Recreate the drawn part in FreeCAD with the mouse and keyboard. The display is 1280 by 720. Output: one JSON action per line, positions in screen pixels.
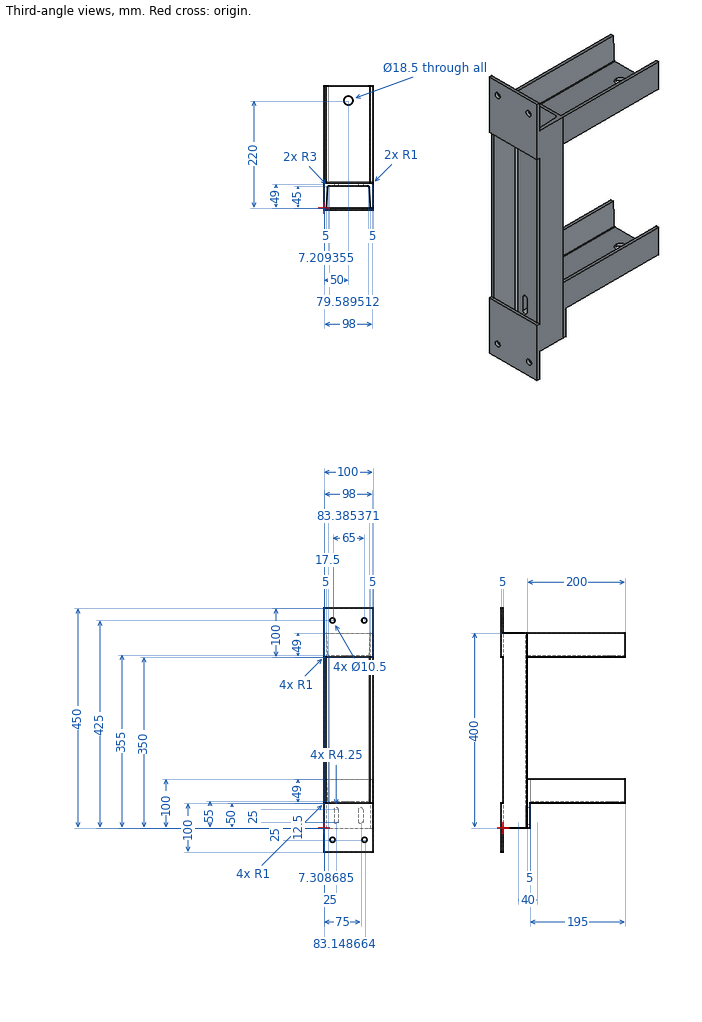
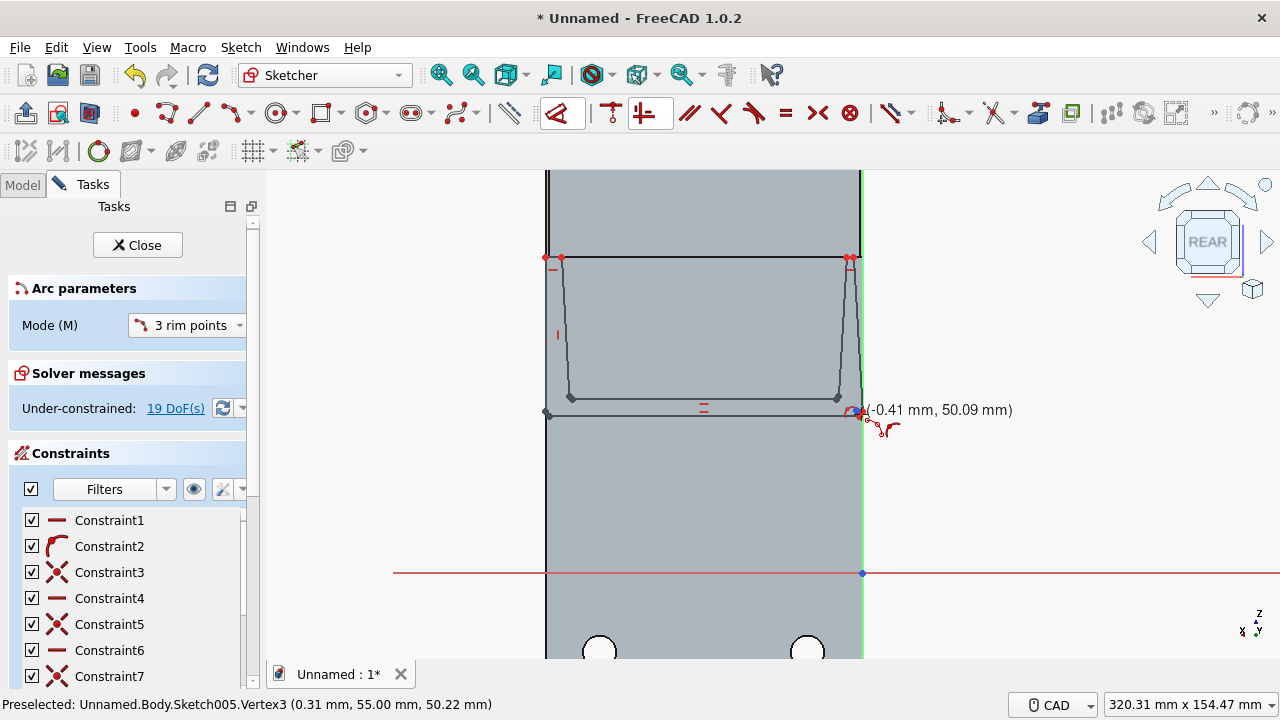
{"action": "scroll", "coordinate": [840, 396], "scroll_direction": "up", "scroll_amount": 7}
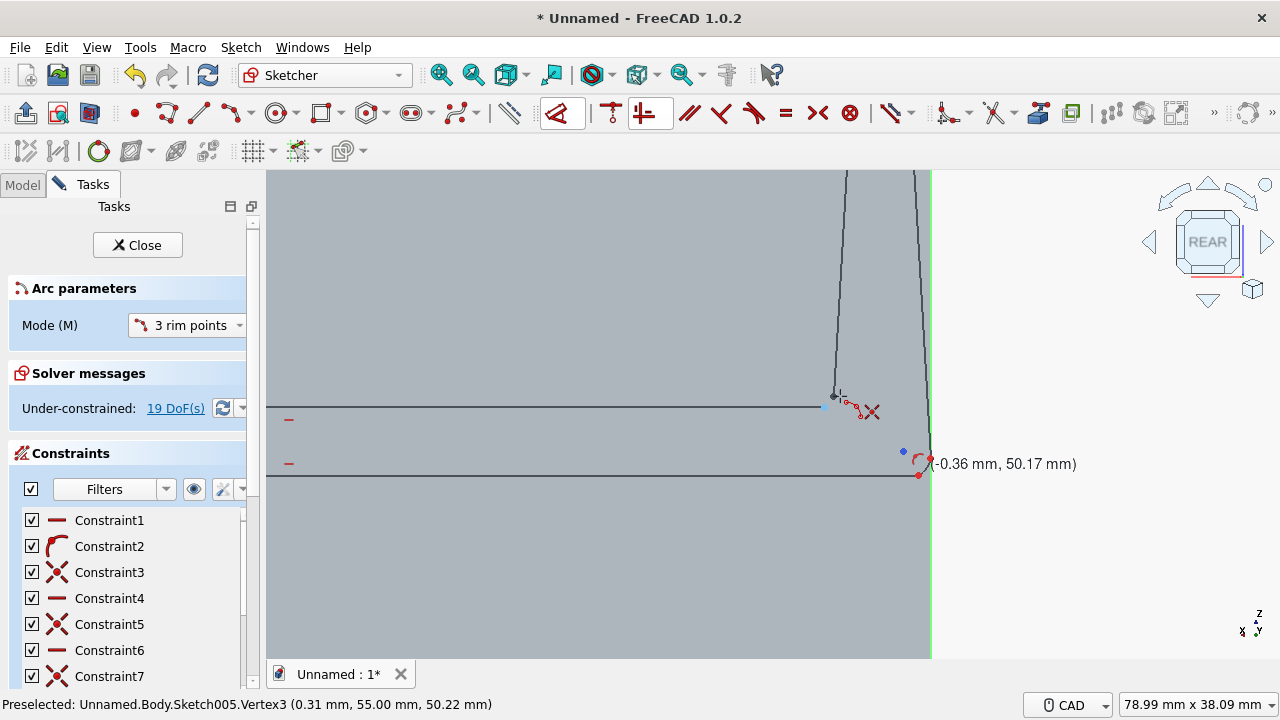
{"action": "left_click", "coordinate": [834, 397]}
{"action": "left_click", "coordinate": [824, 407]}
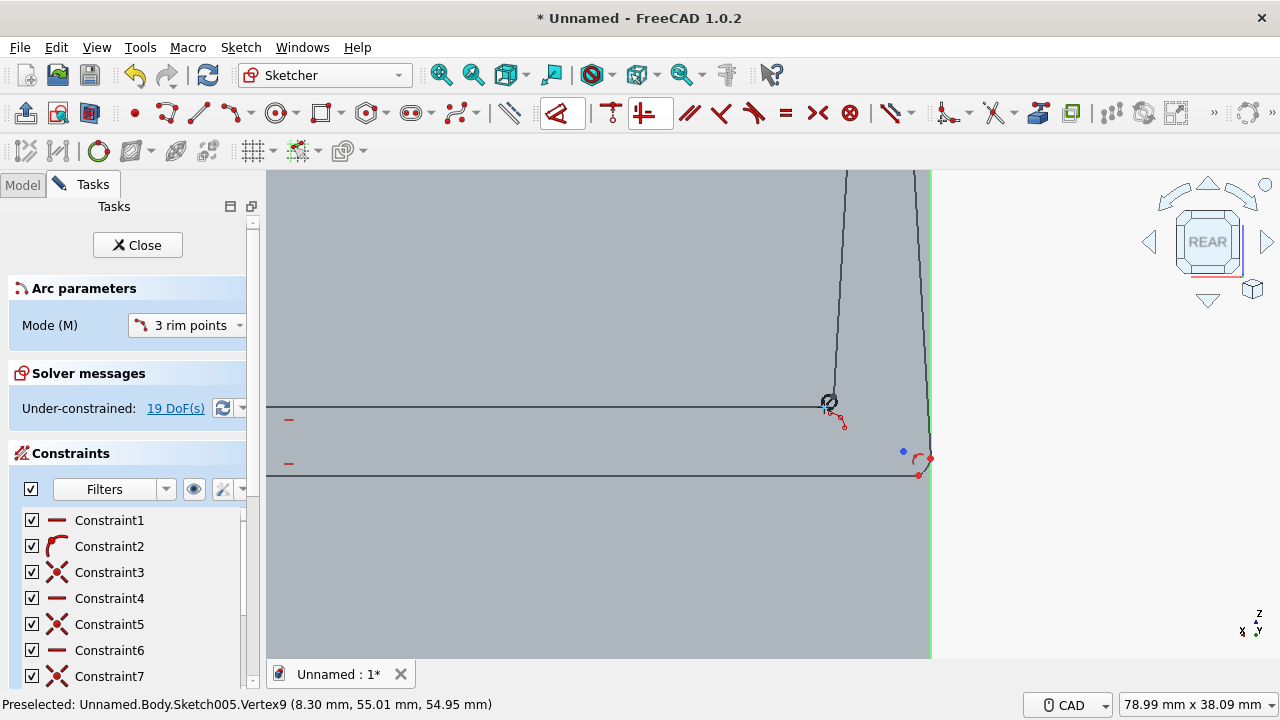
{"action": "scroll", "coordinate": [833, 403], "scroll_direction": "up", "scroll_amount": 8}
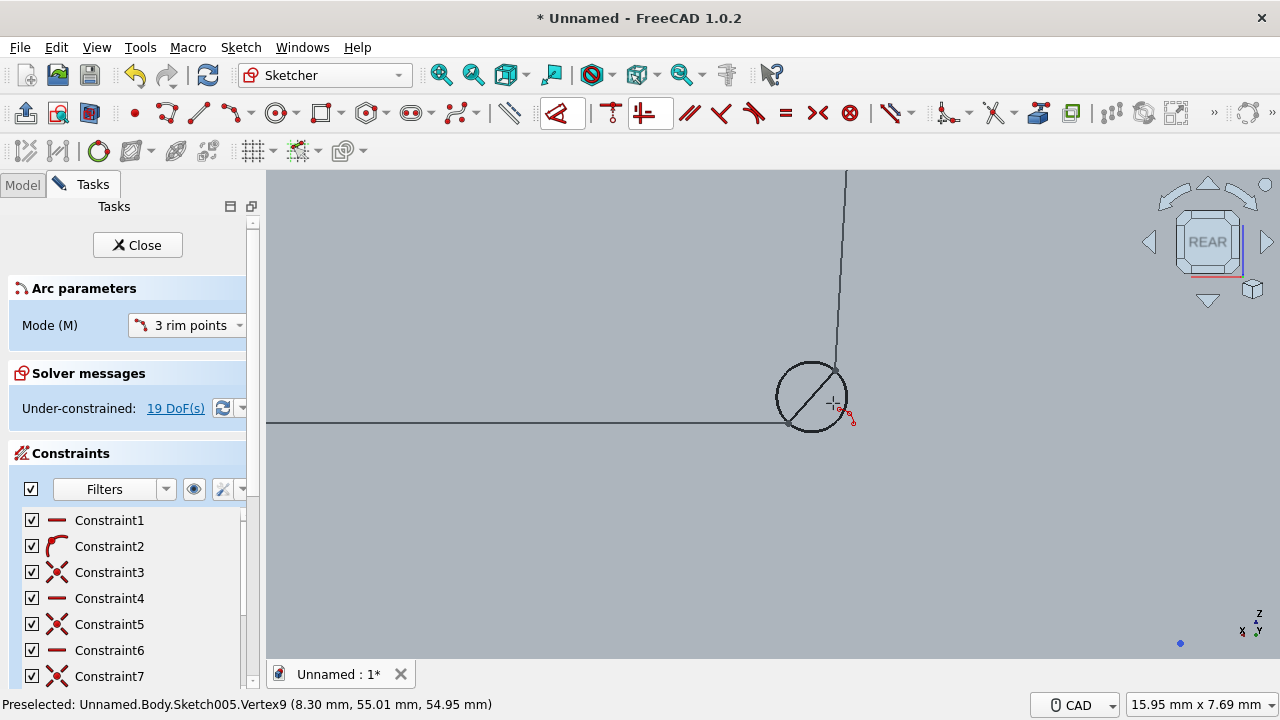
{"action": "left_click", "coordinate": [832, 402]}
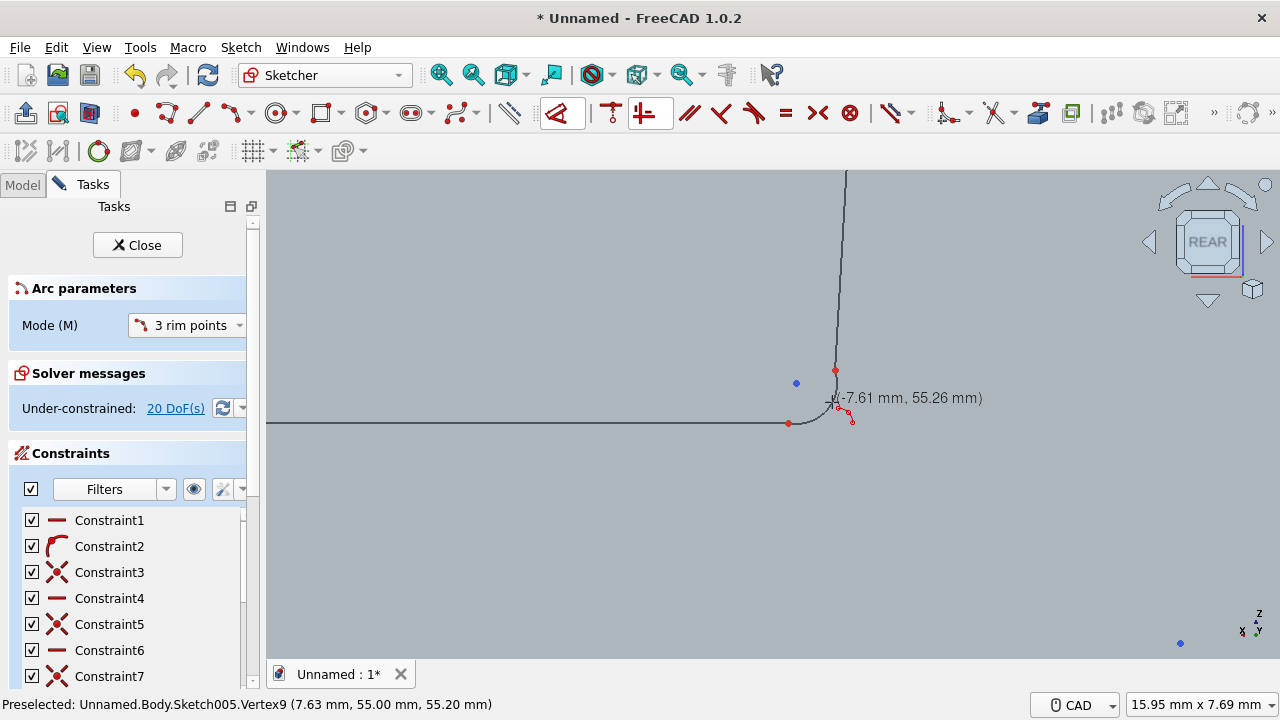
{"action": "scroll", "coordinate": [839, 398], "scroll_direction": "down", "scroll_amount": 15}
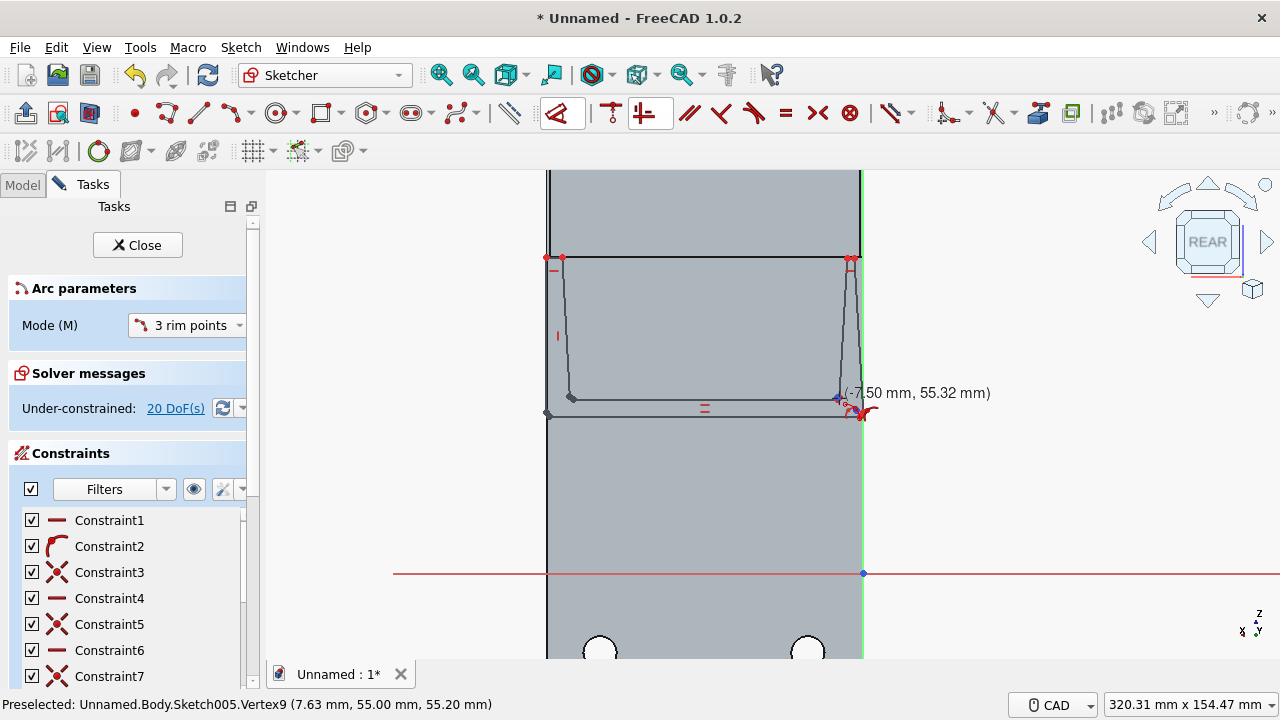
{"action": "scroll", "coordinate": [573, 400], "scroll_direction": "up", "scroll_amount": 7}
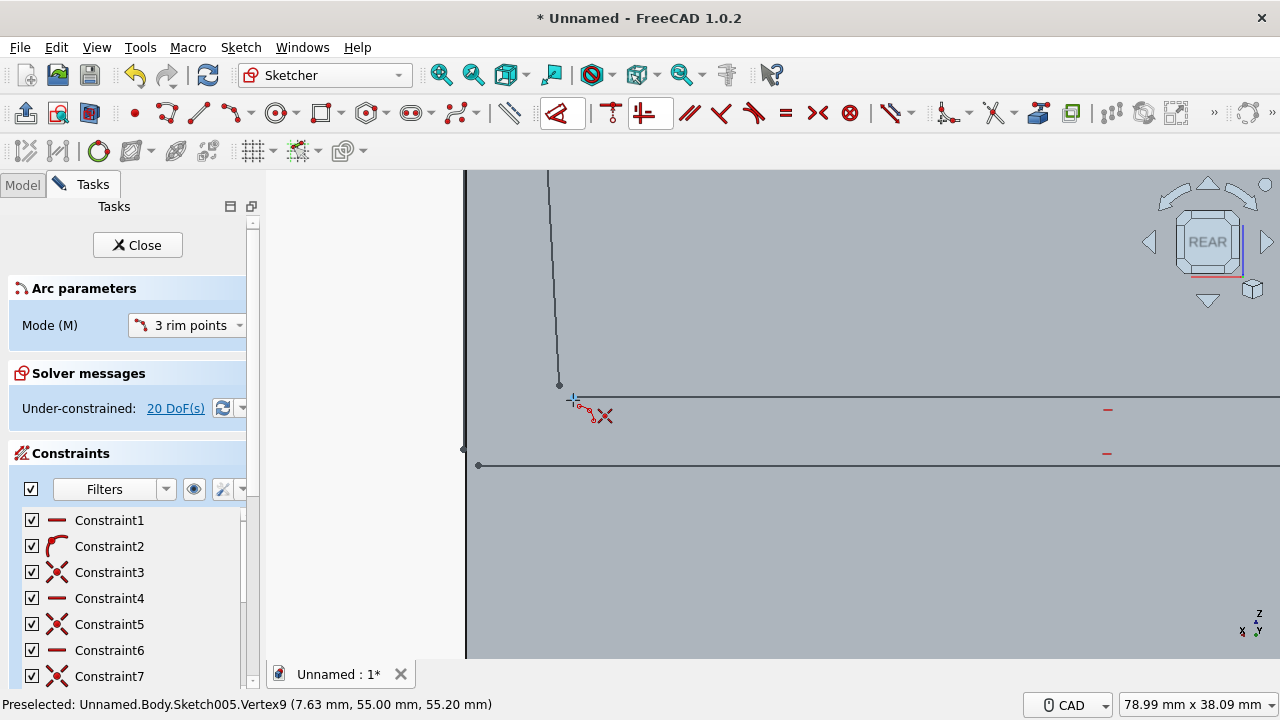
{"action": "left_click", "coordinate": [573, 397]}
{"action": "left_click", "coordinate": [559, 385]}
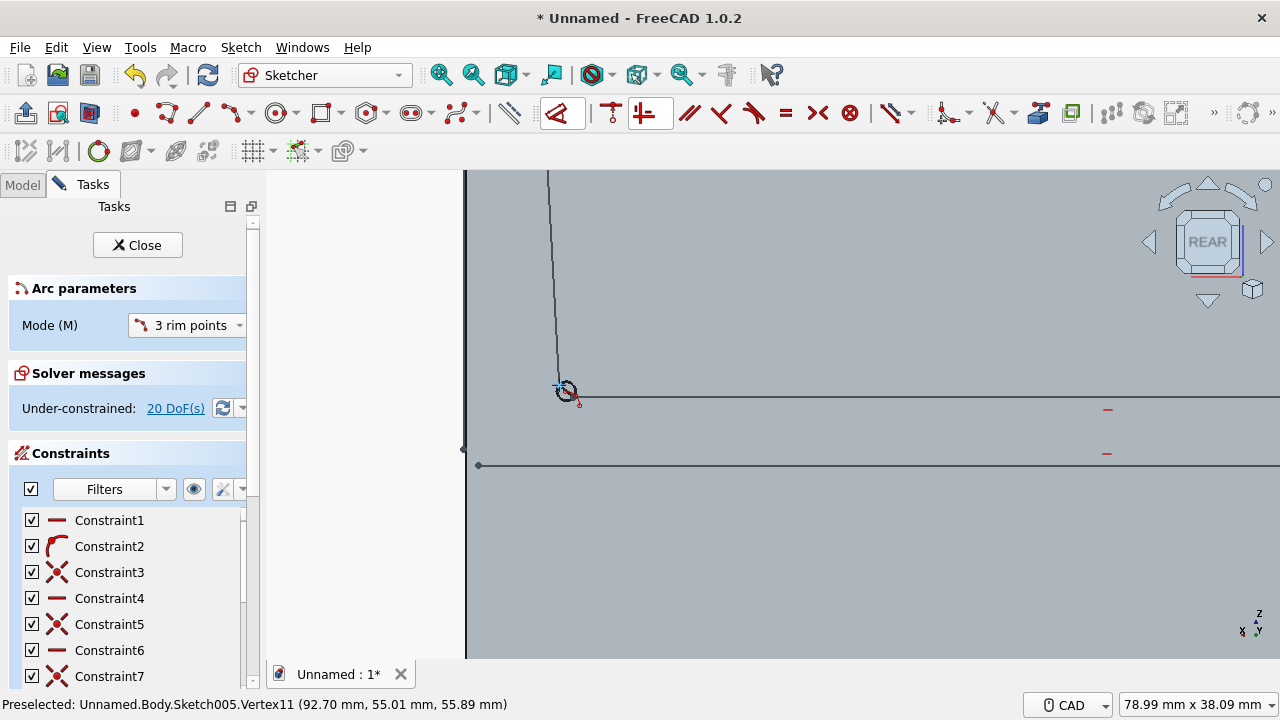
{"action": "scroll", "coordinate": [563, 393], "scroll_direction": "up", "scroll_amount": 8}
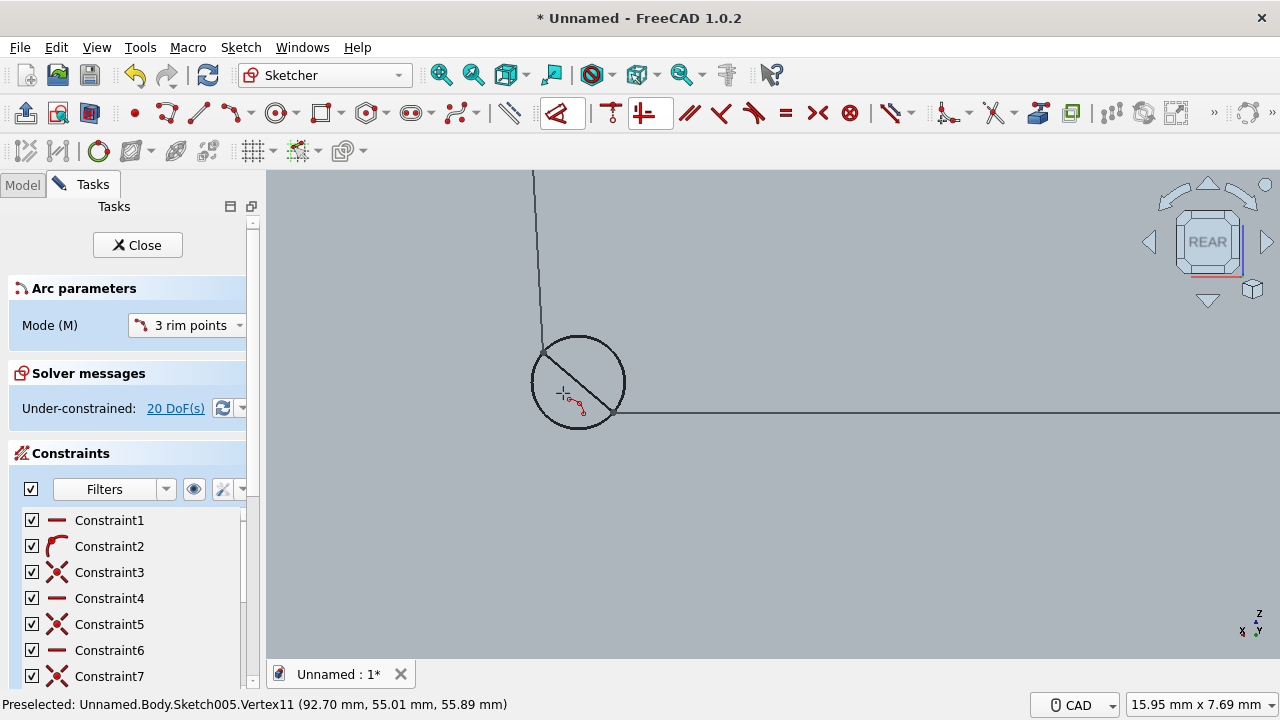
{"action": "left_click", "coordinate": [564, 392]}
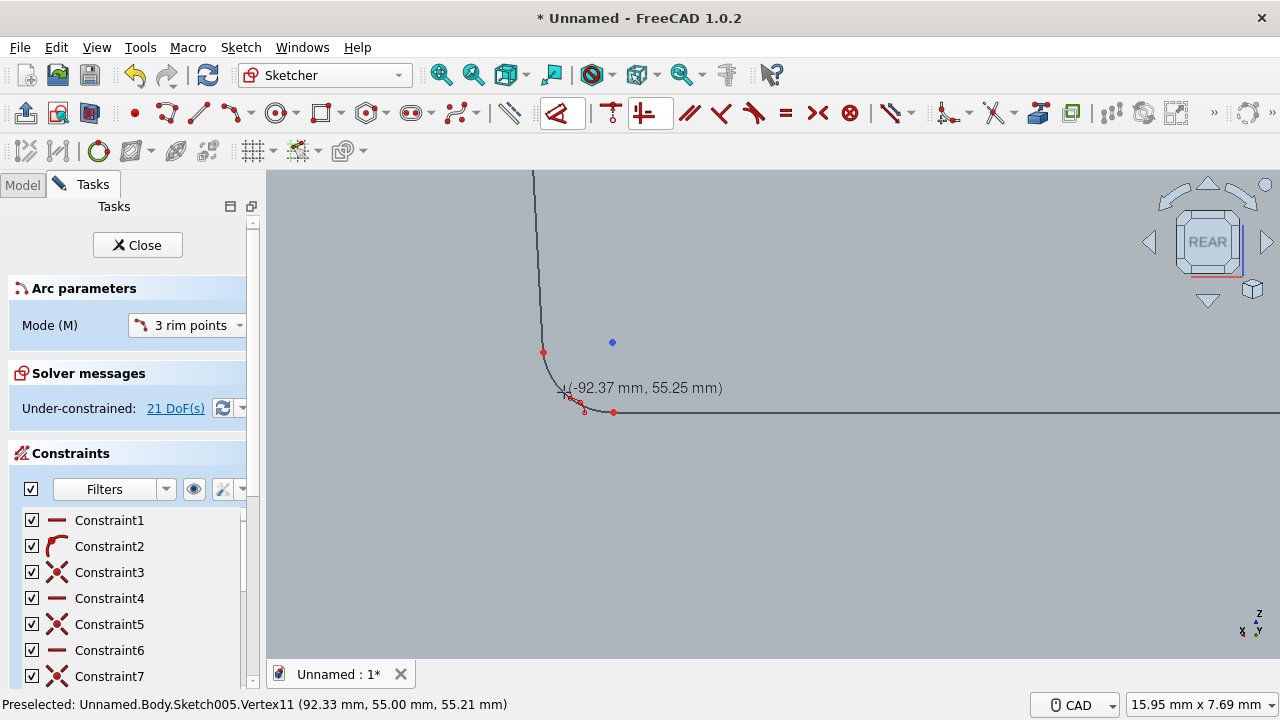
{"action": "scroll", "coordinate": [571, 398], "scroll_direction": "down", "scroll_amount": 15}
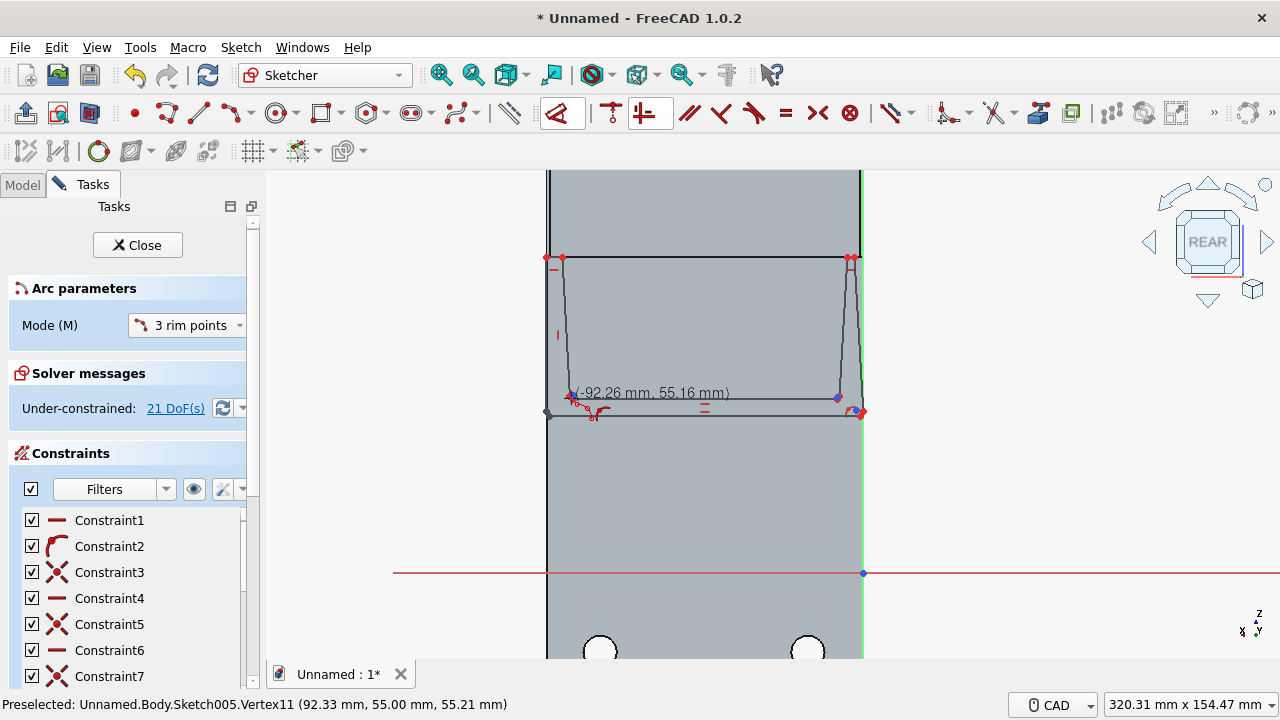
{"action": "scroll", "coordinate": [547, 412], "scroll_direction": "up", "scroll_amount": 7}